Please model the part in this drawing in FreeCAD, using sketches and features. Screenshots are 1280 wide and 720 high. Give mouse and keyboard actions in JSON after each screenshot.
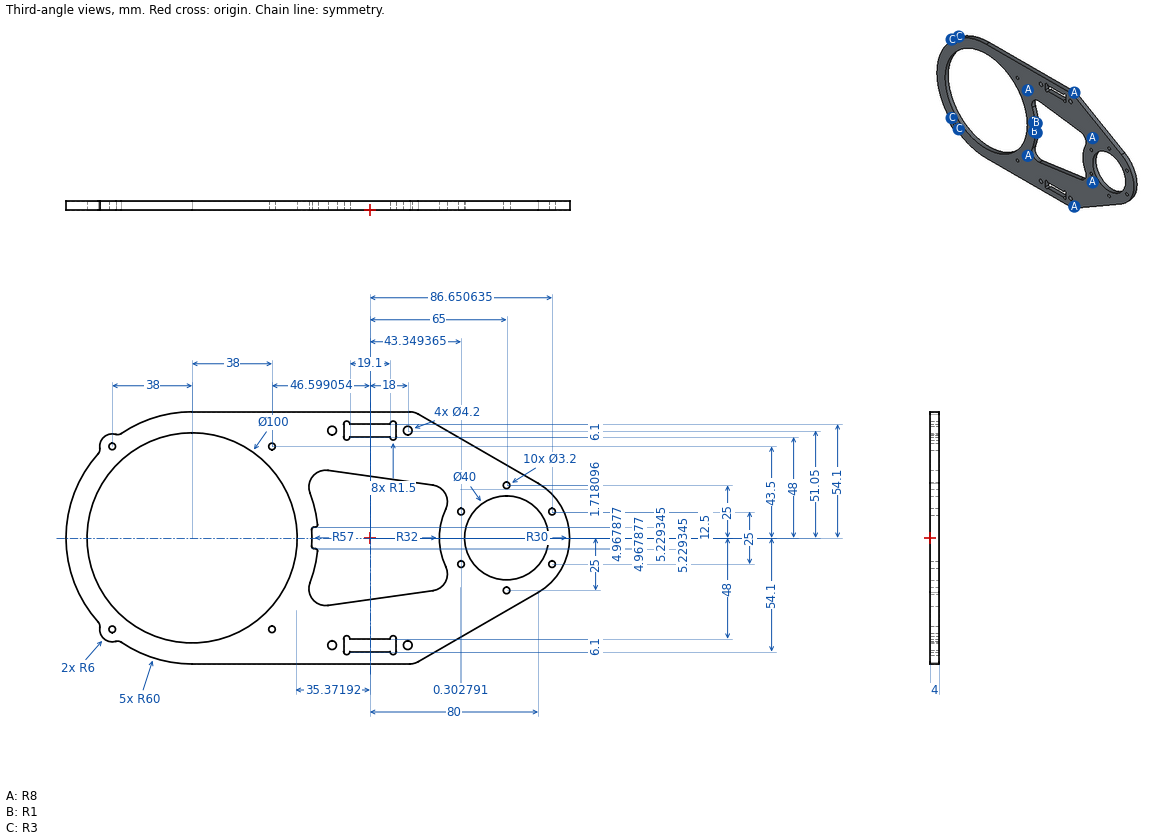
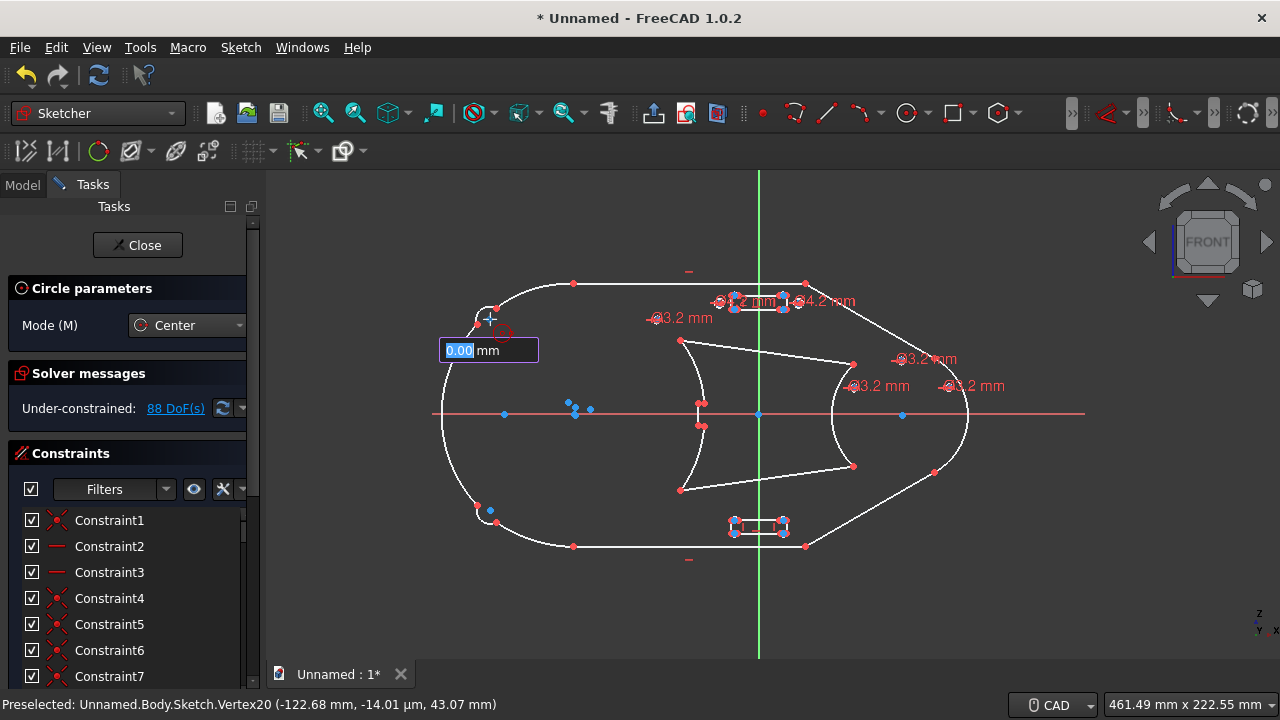
{"action": "scroll", "coordinate": [493, 318], "scroll_direction": "up", "scroll_amount": 8}
{"action": "mouse_move", "coordinate": [492, 315]}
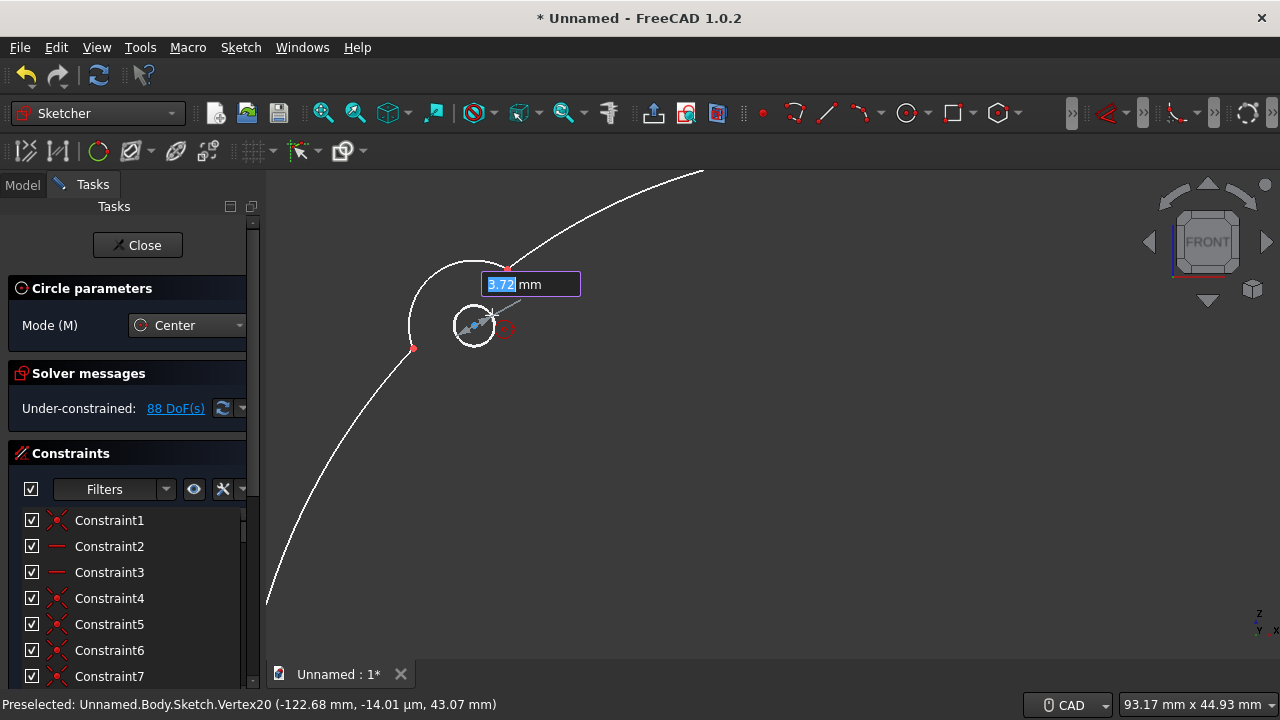
{"action": "type", "text": "3.2"}
{"action": "key", "text": "Return"}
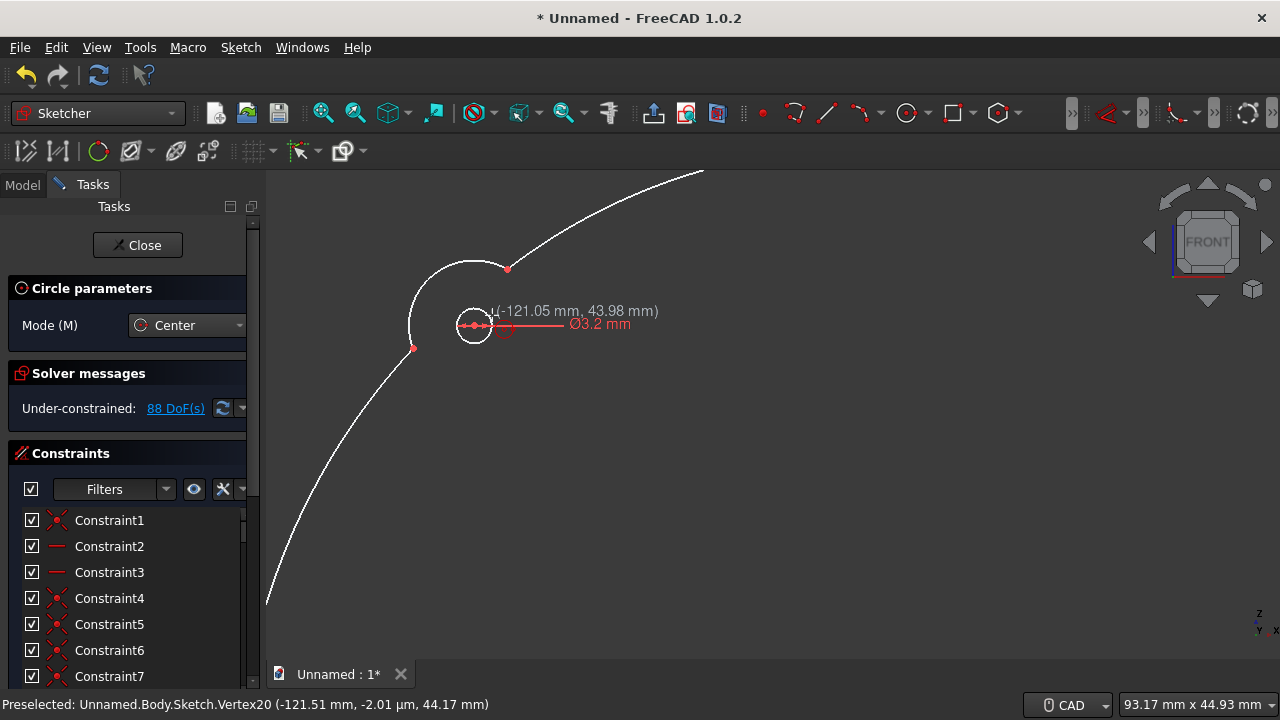
{"action": "scroll", "coordinate": [493, 318], "scroll_direction": "down", "scroll_amount": 8}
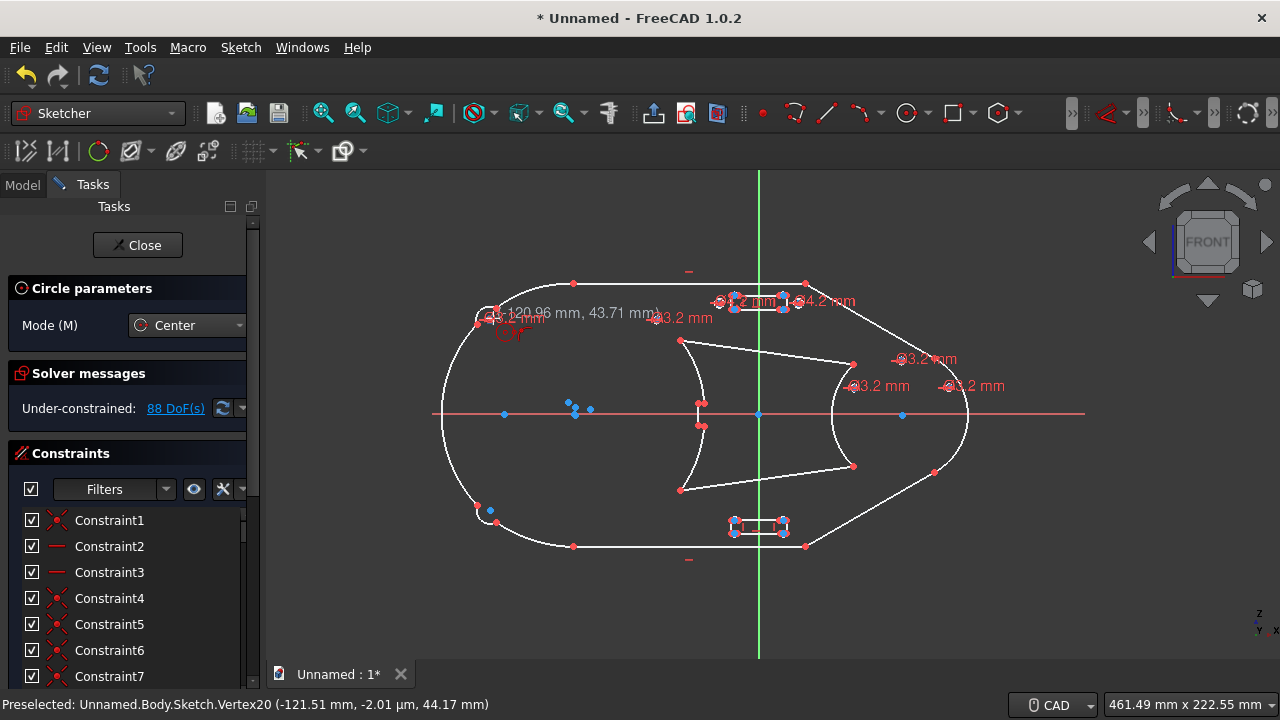
{"action": "left_click", "coordinate": [902, 414]}
{"action": "mouse_move", "coordinate": [933, 446]}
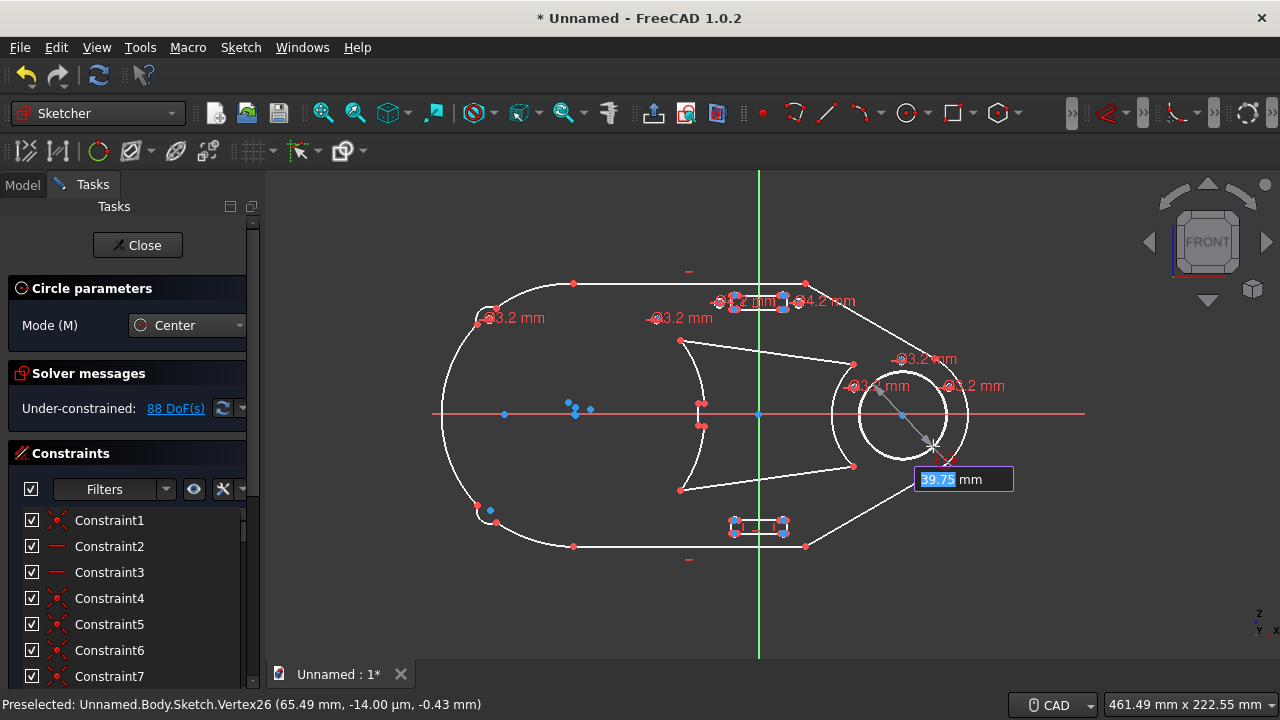
{"action": "type", "text": "40"}
{"action": "key", "text": "Return"}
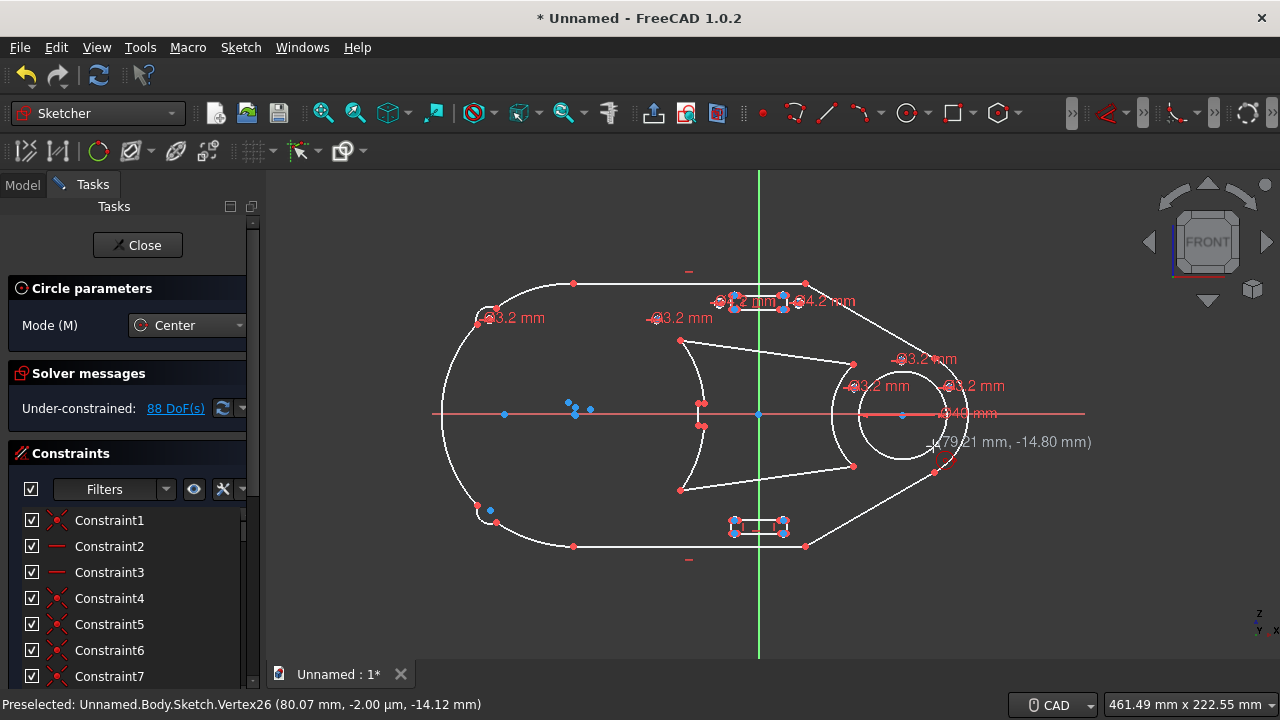
{"action": "scroll", "coordinate": [949, 442], "scroll_direction": "up", "scroll_amount": 10}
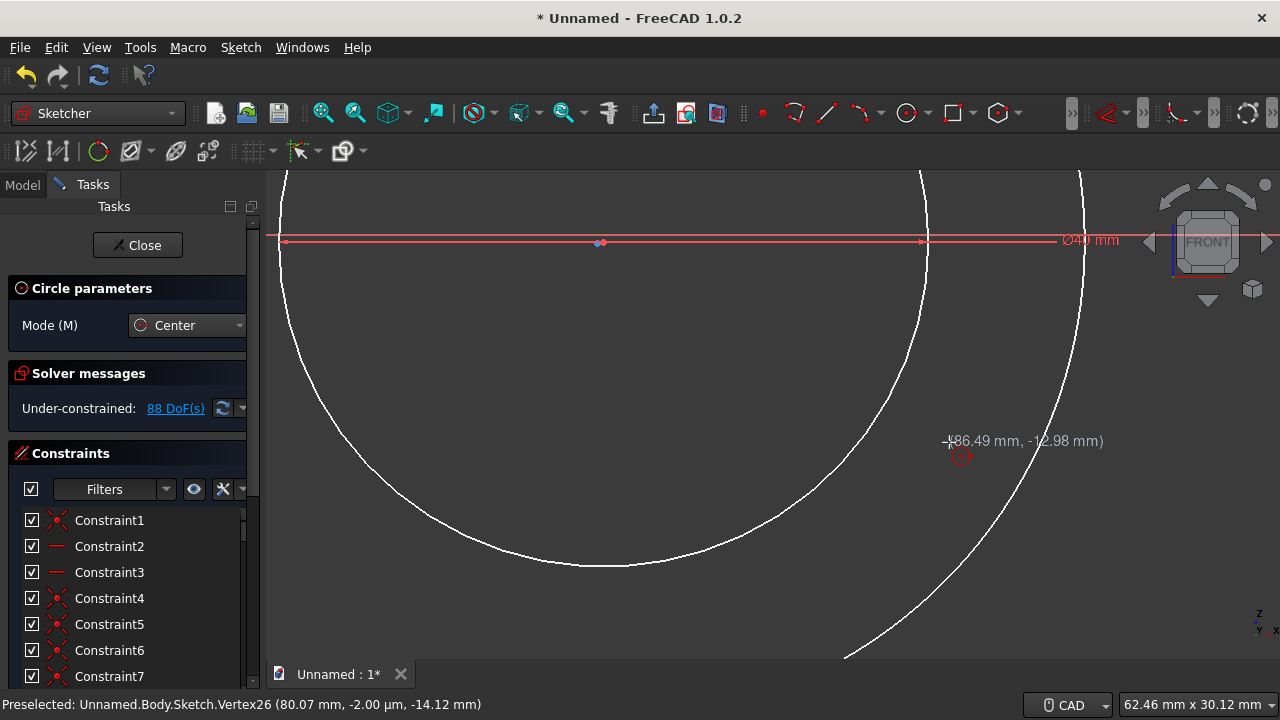
{"action": "scroll", "coordinate": [950, 443], "scroll_direction": "down", "scroll_amount": 10}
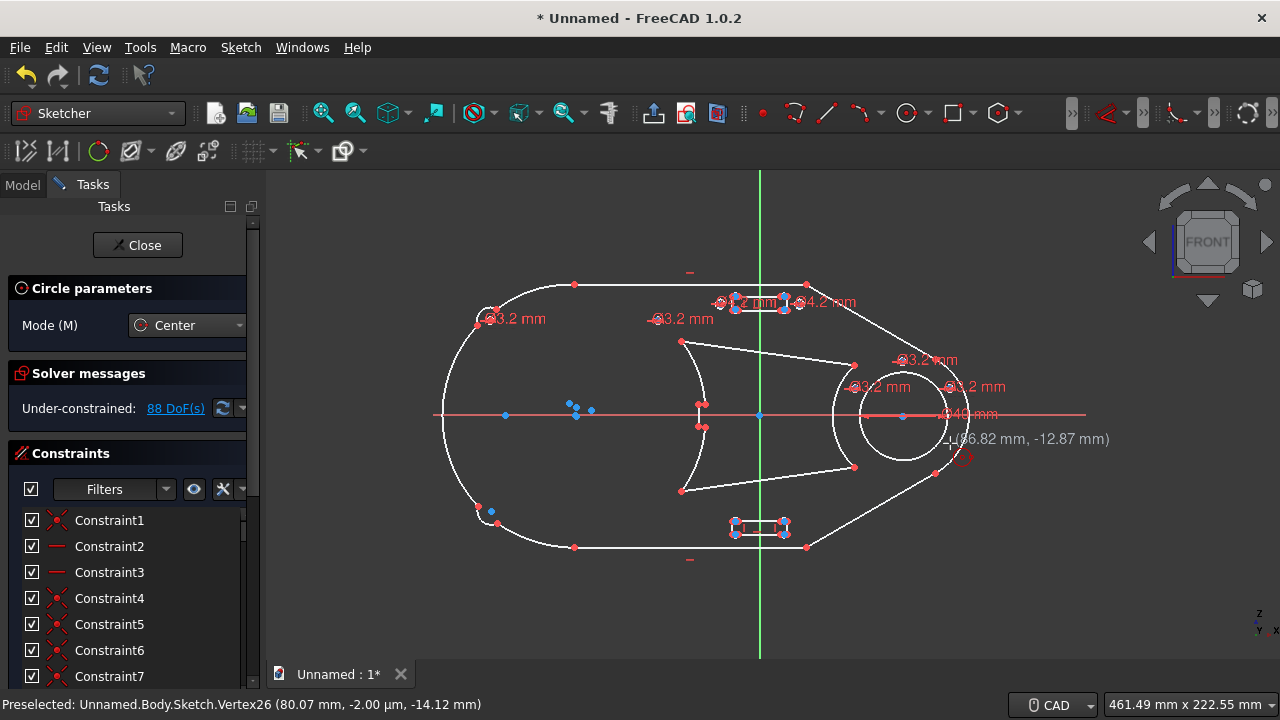
{"action": "scroll", "coordinate": [950, 443], "scroll_direction": "up", "scroll_amount": 2}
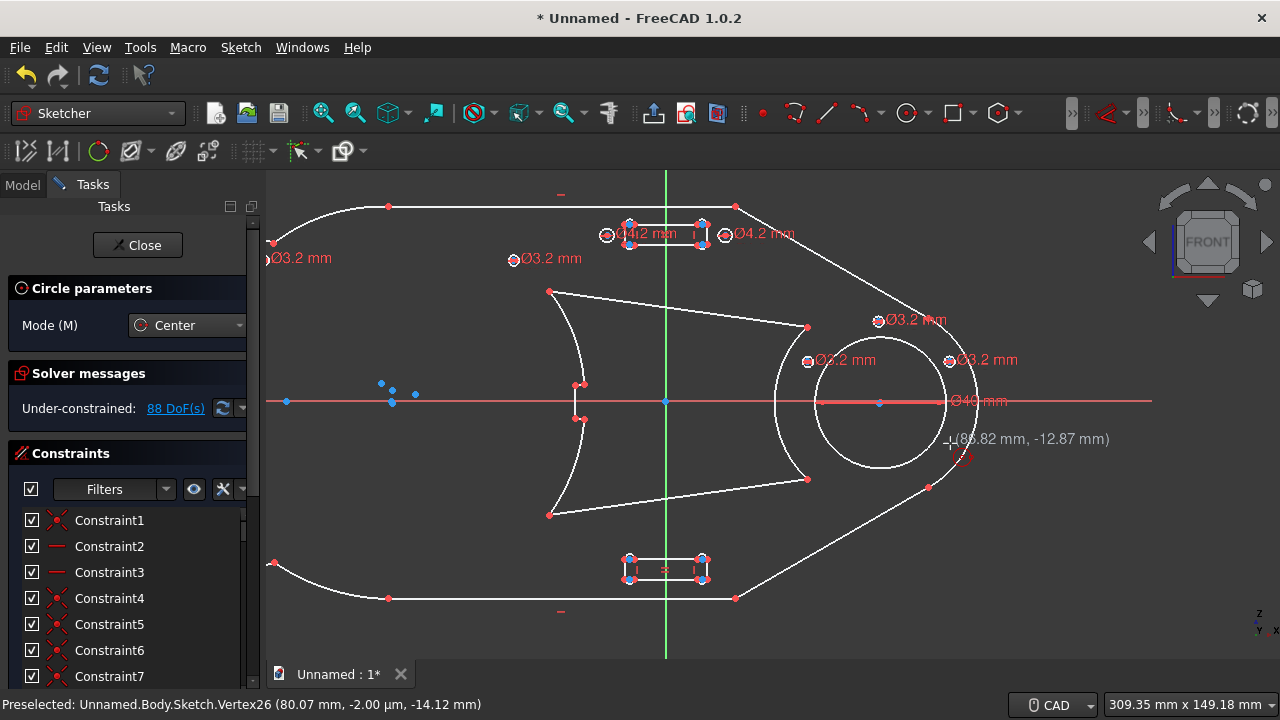
{"action": "left_click", "coordinate": [950, 442]}
{"action": "mouse_move", "coordinate": [954, 439]}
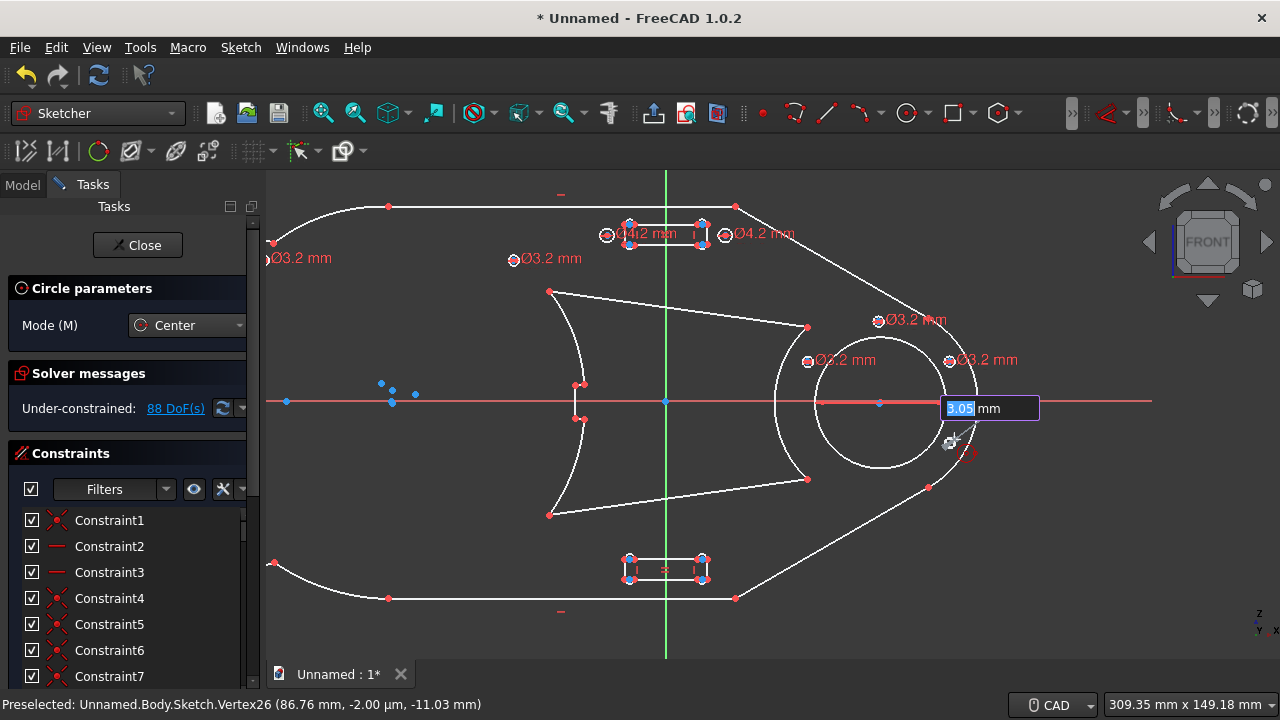
{"action": "type", "text": "3.2"}
{"action": "key", "text": "Return"}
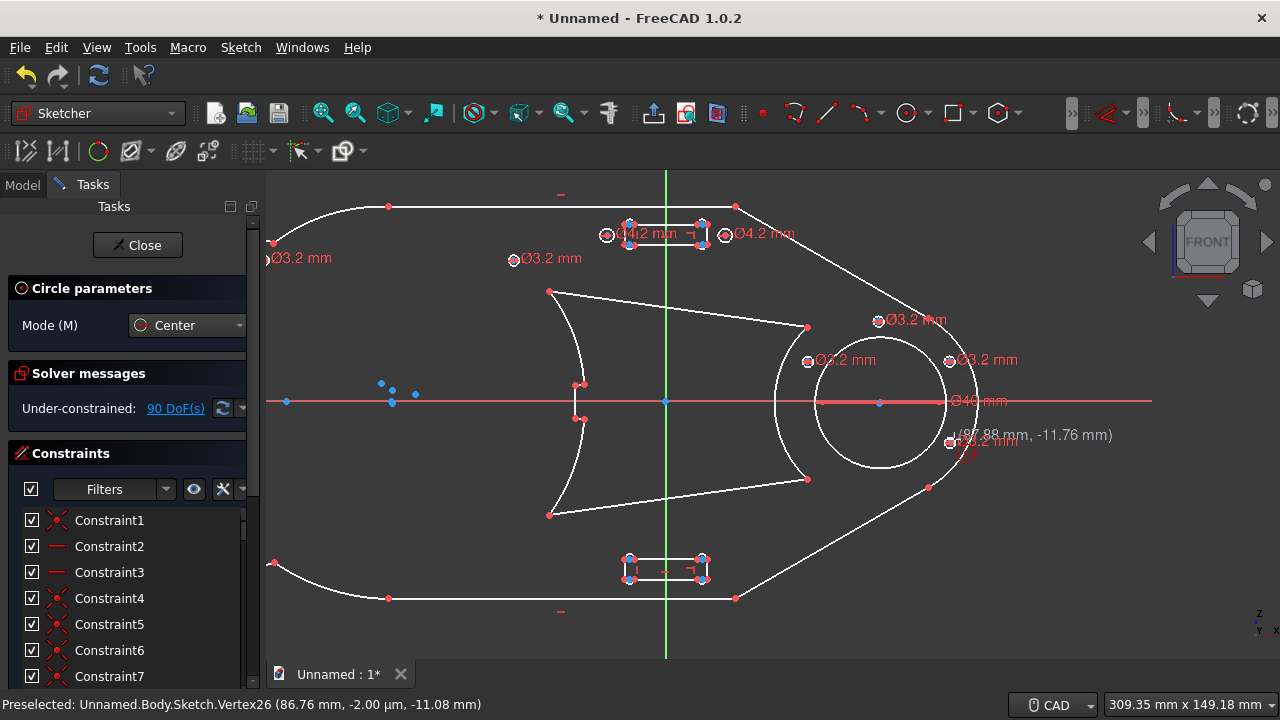
{"action": "scroll", "coordinate": [808, 442], "scroll_direction": "up", "scroll_amount": 8}